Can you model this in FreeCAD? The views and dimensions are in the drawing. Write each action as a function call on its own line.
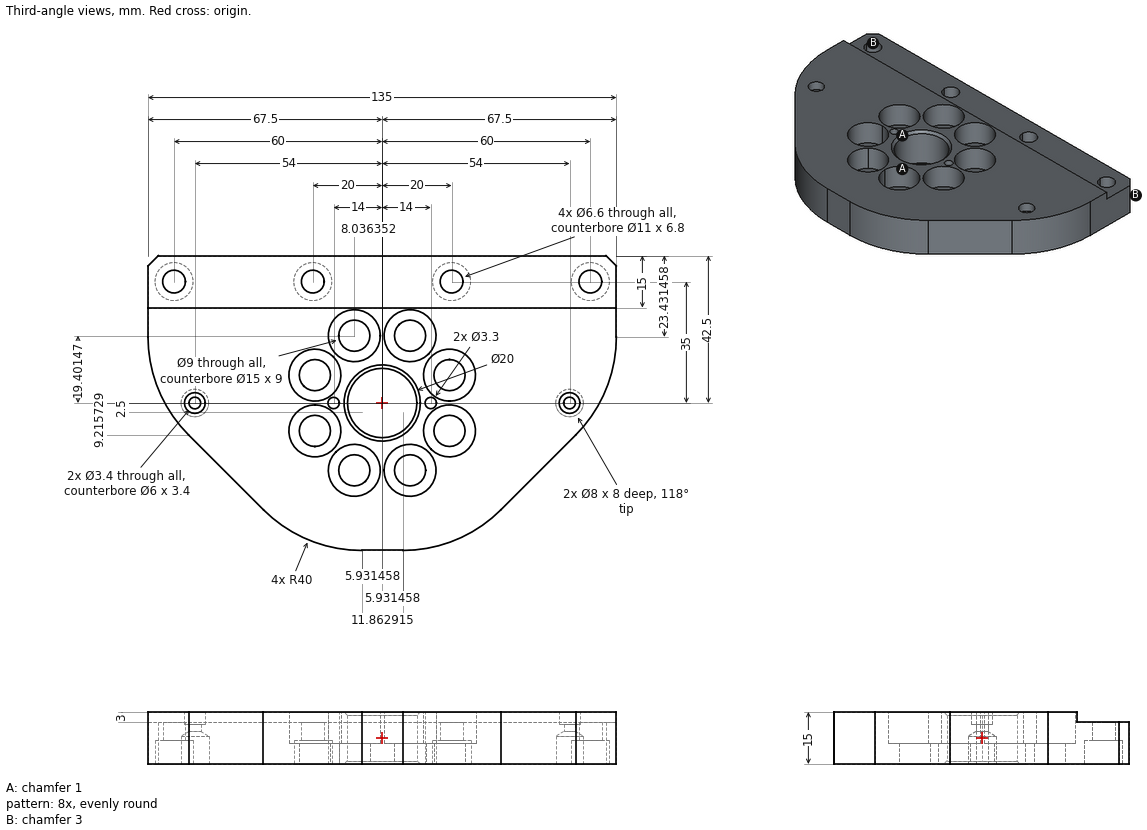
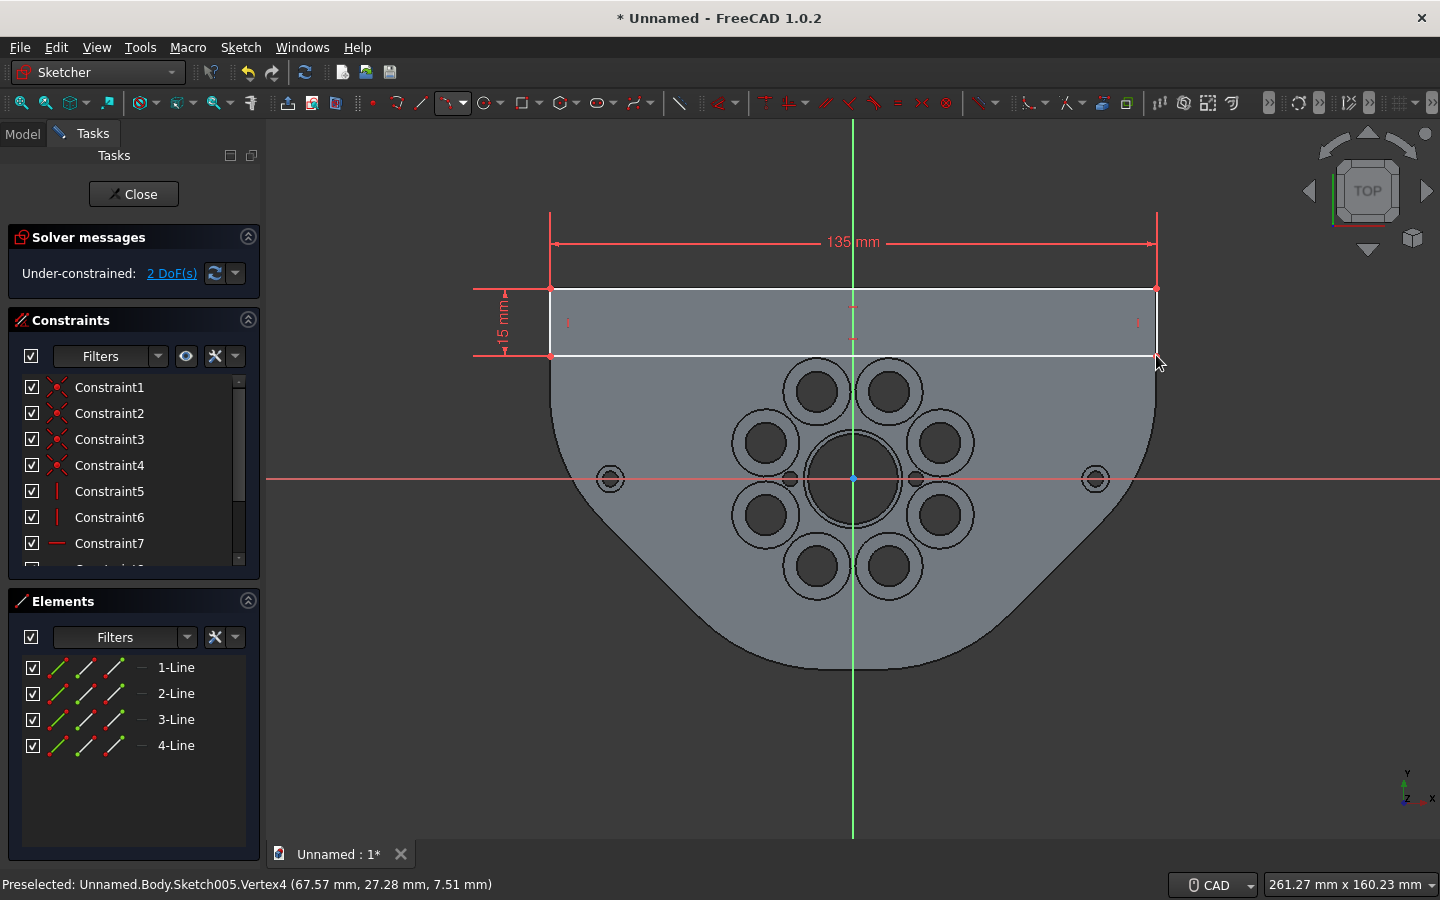
click(718, 104)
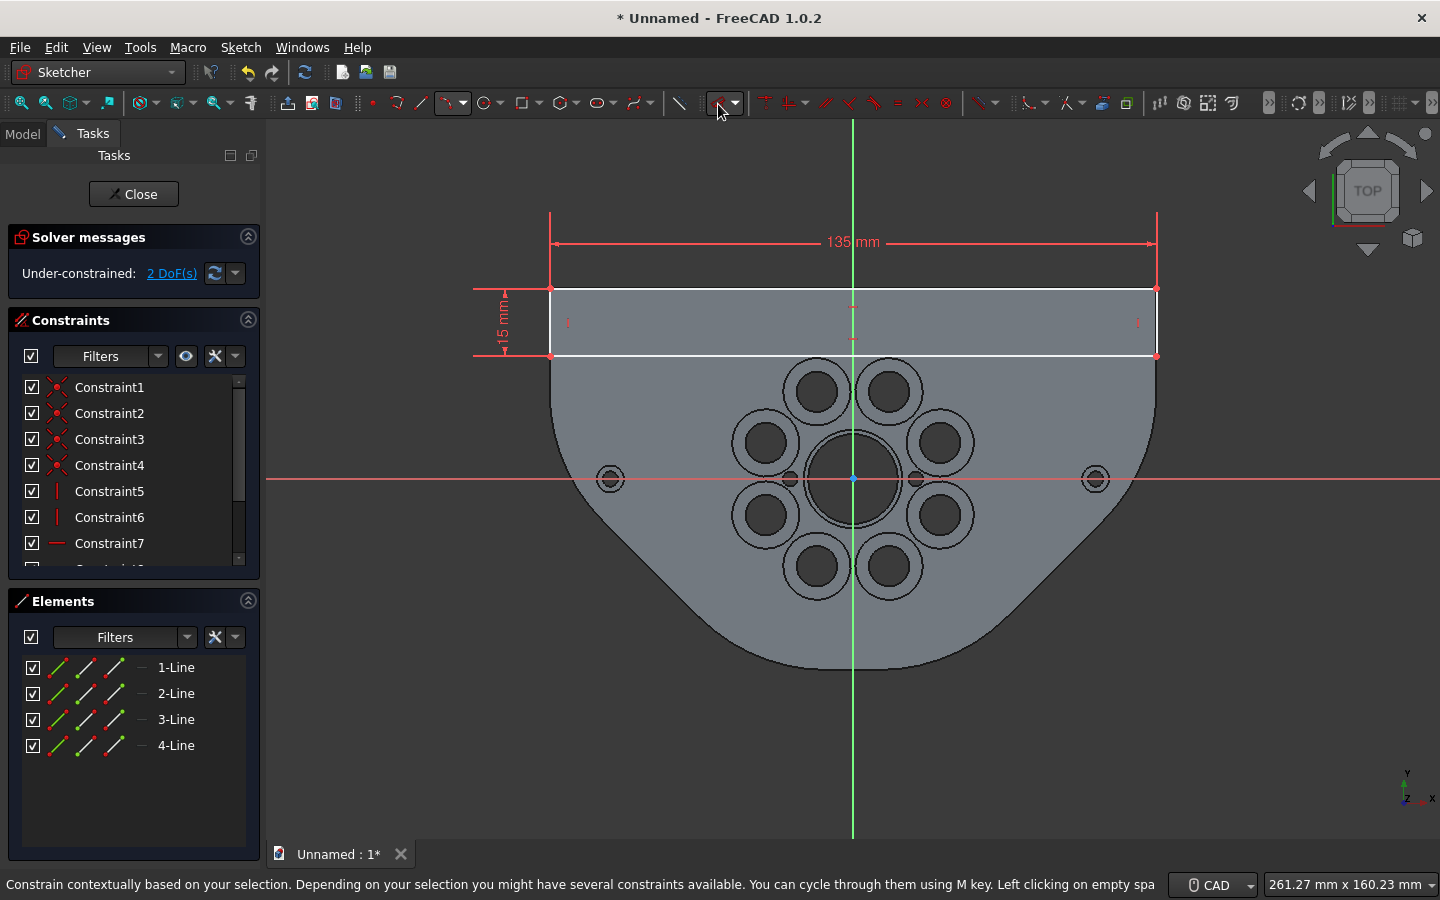
click(550, 289)
click(702, 513)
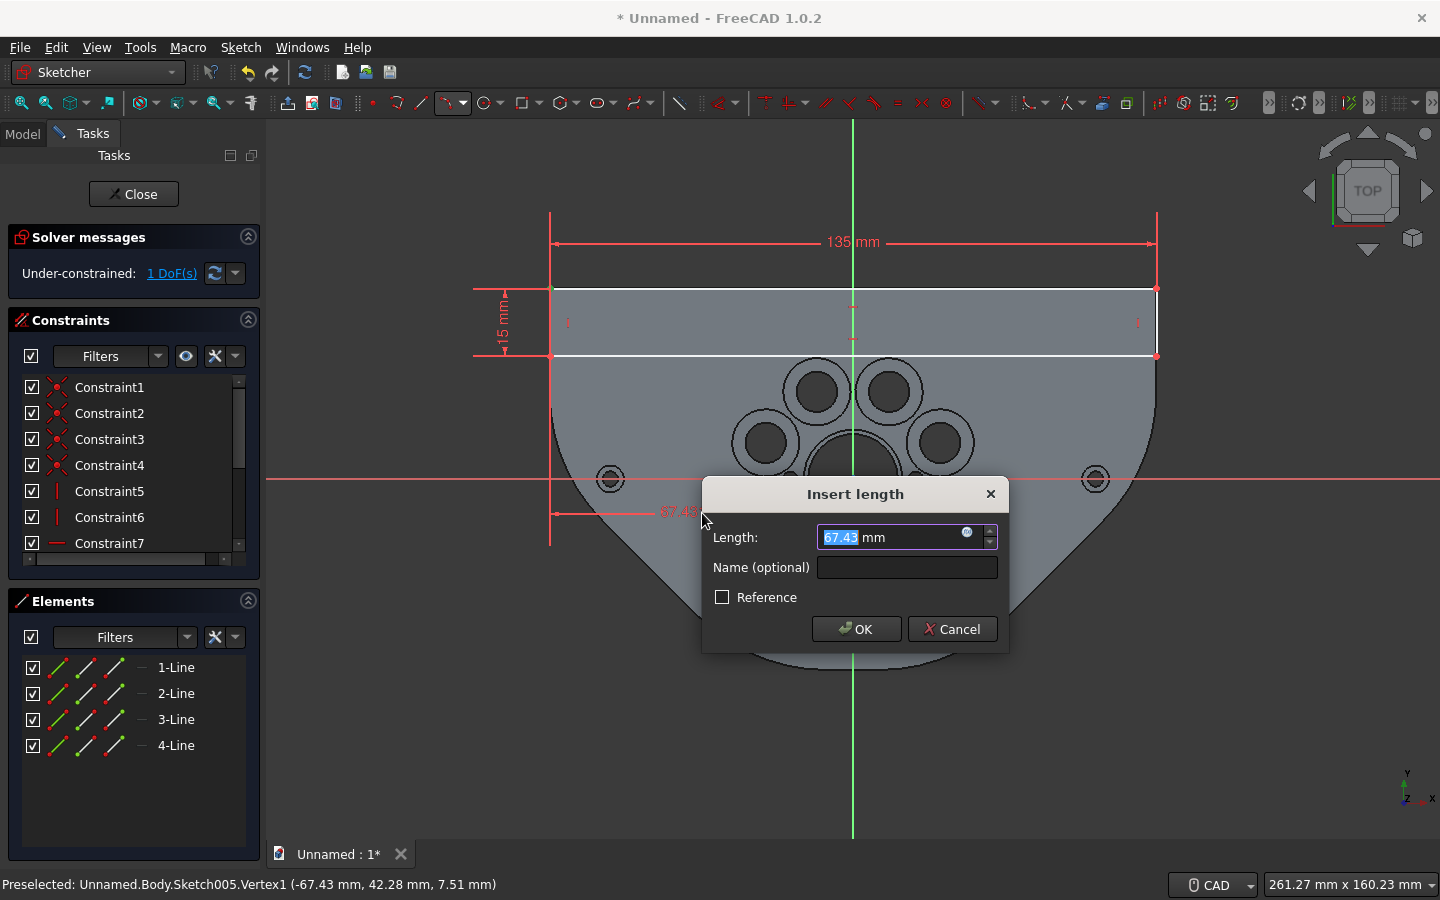
text(67.5)
key(Return)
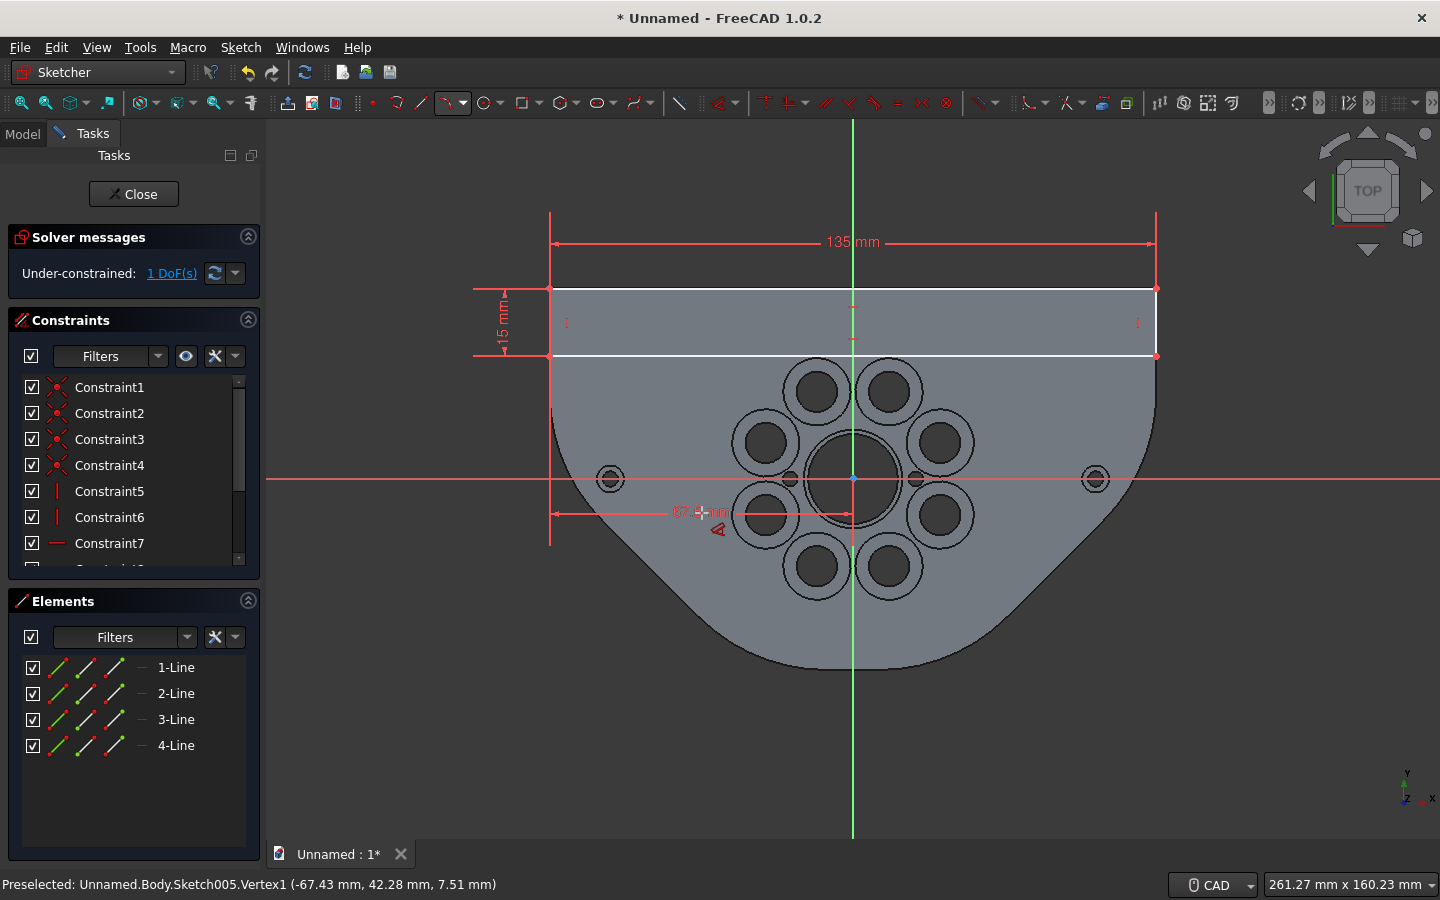
click(550, 289)
click(516, 384)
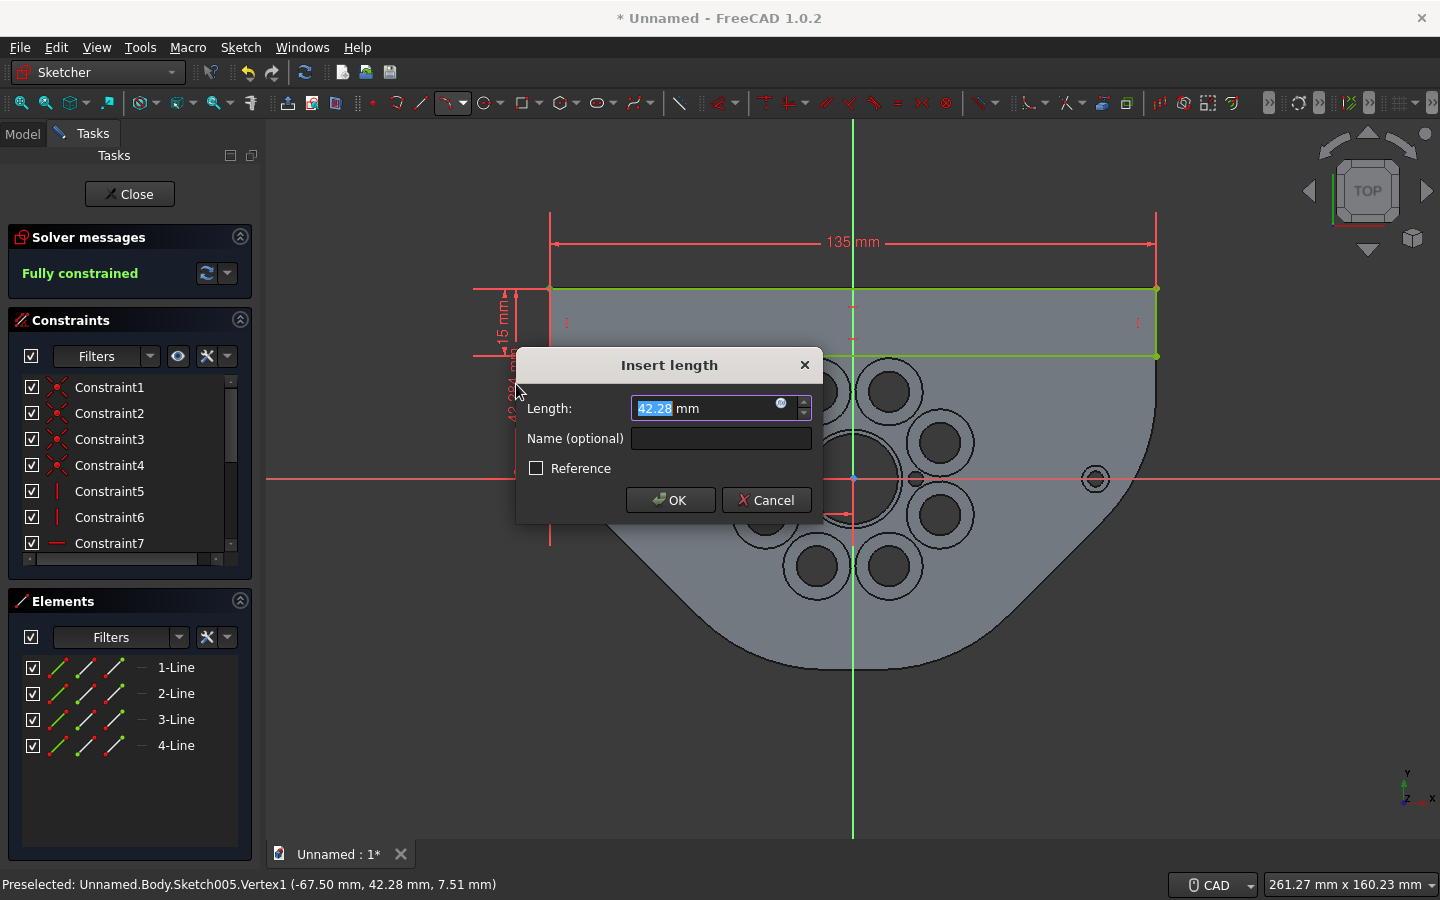
text(42.5)
key(Return)
key(Escape)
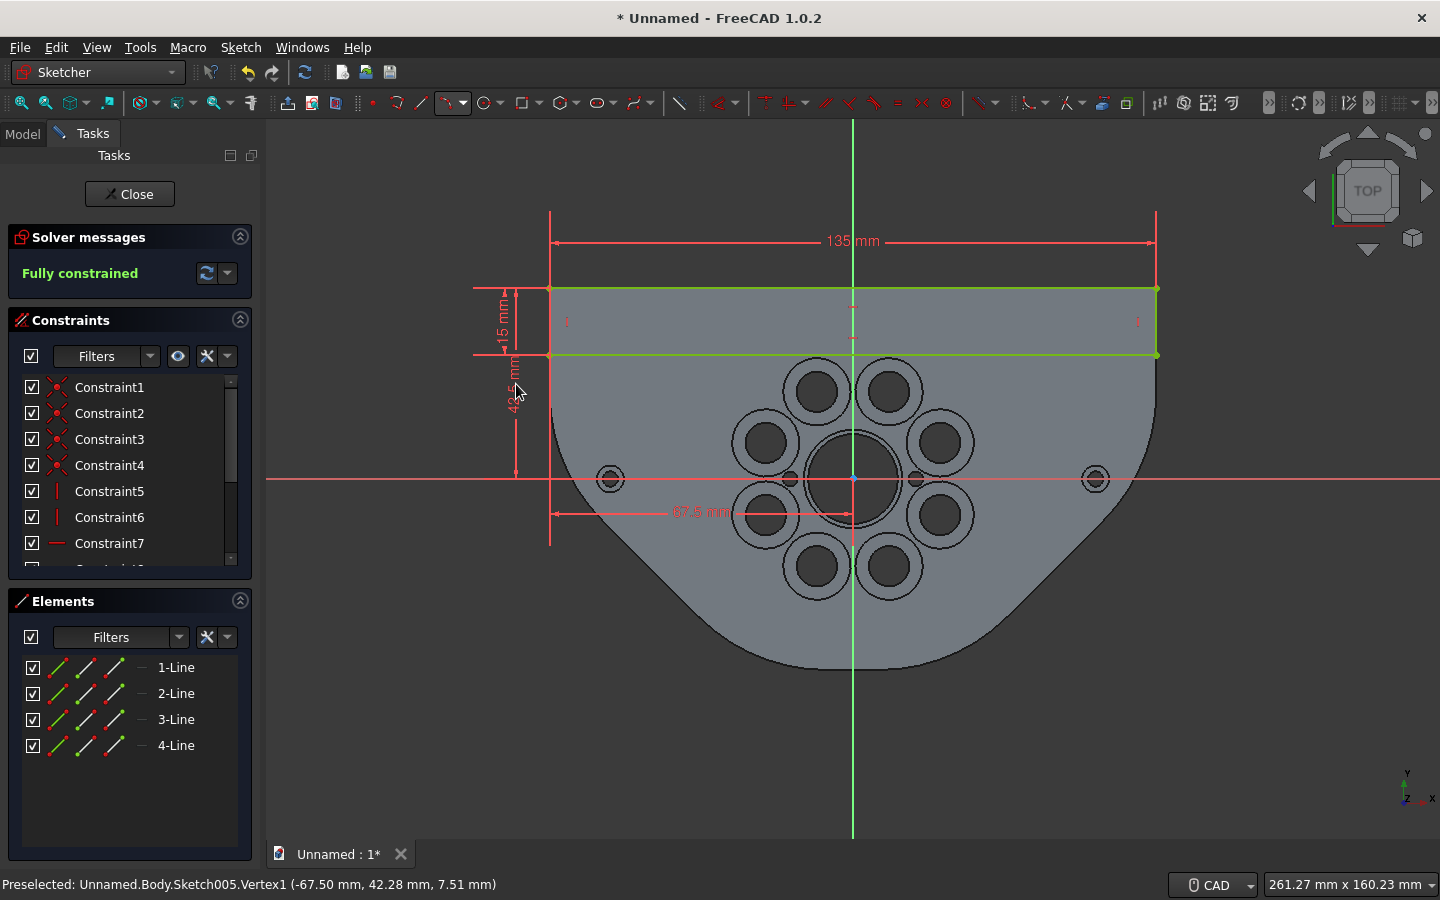
click(130, 194)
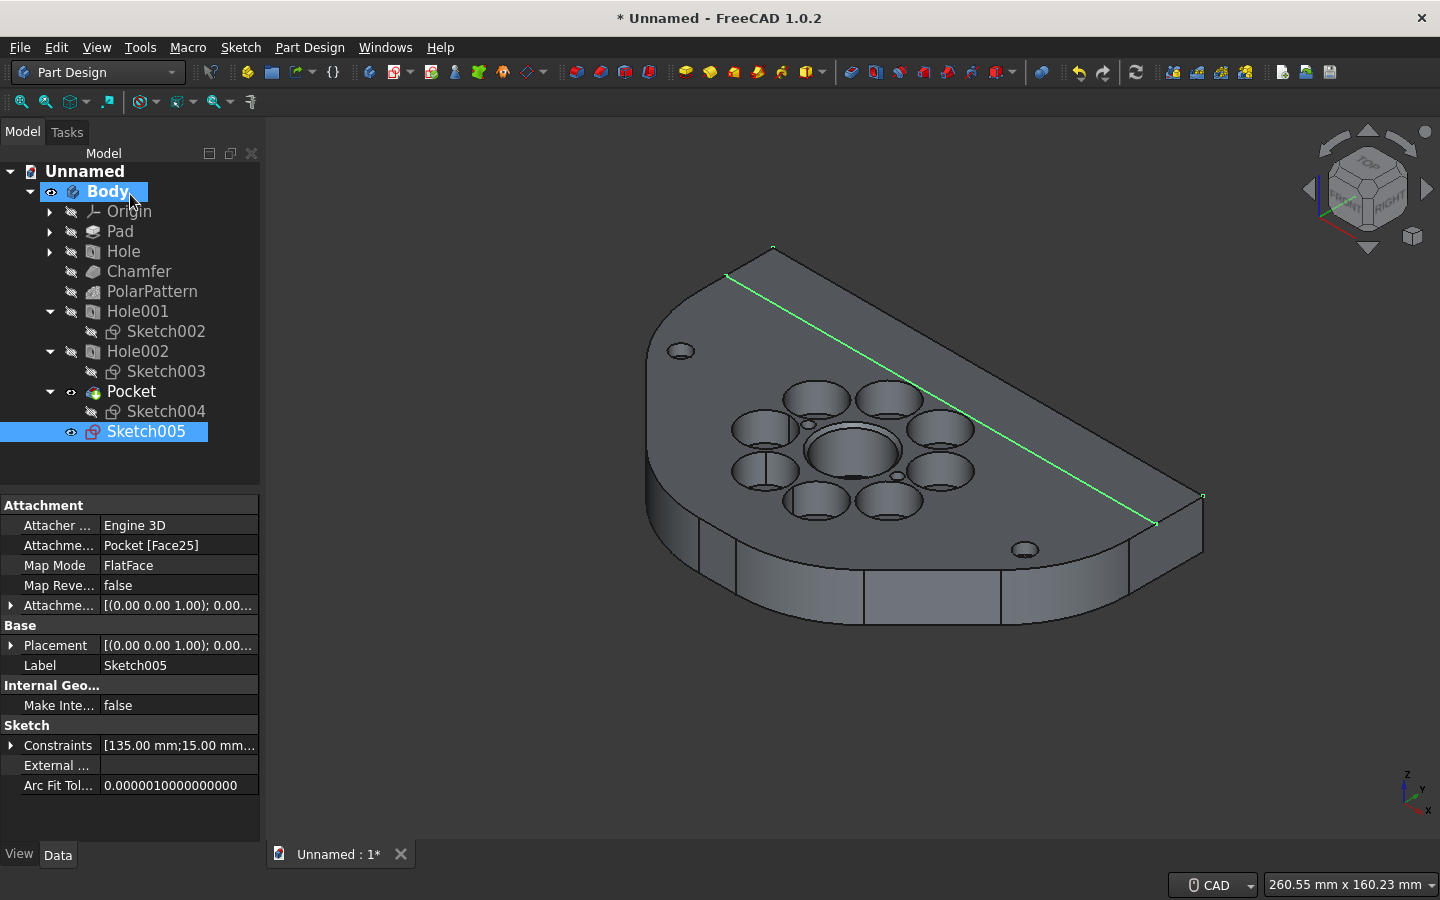
click(852, 72)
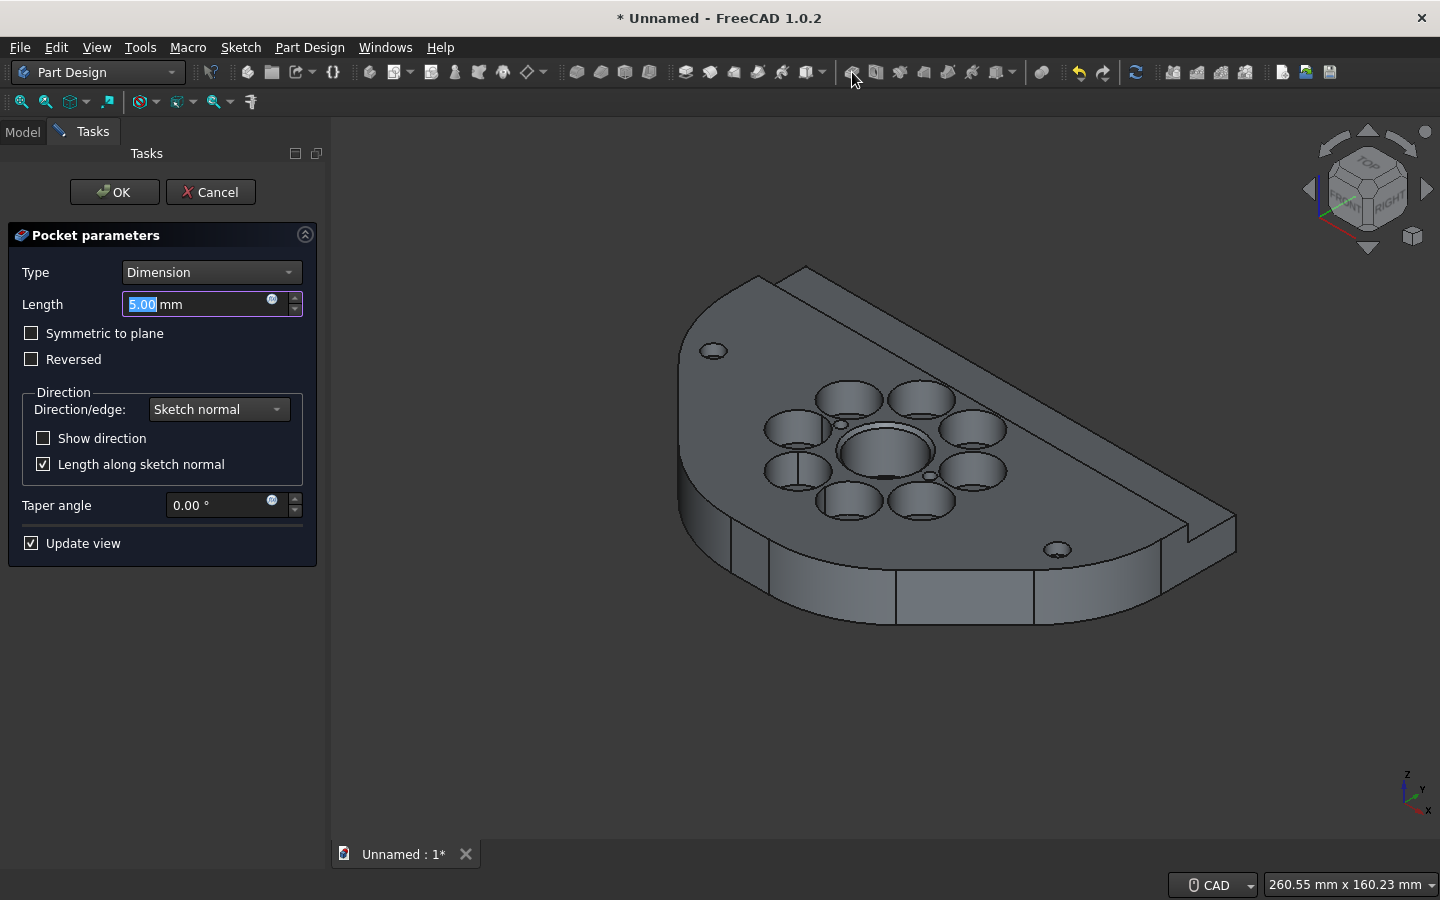
text(3)
key(Tab)